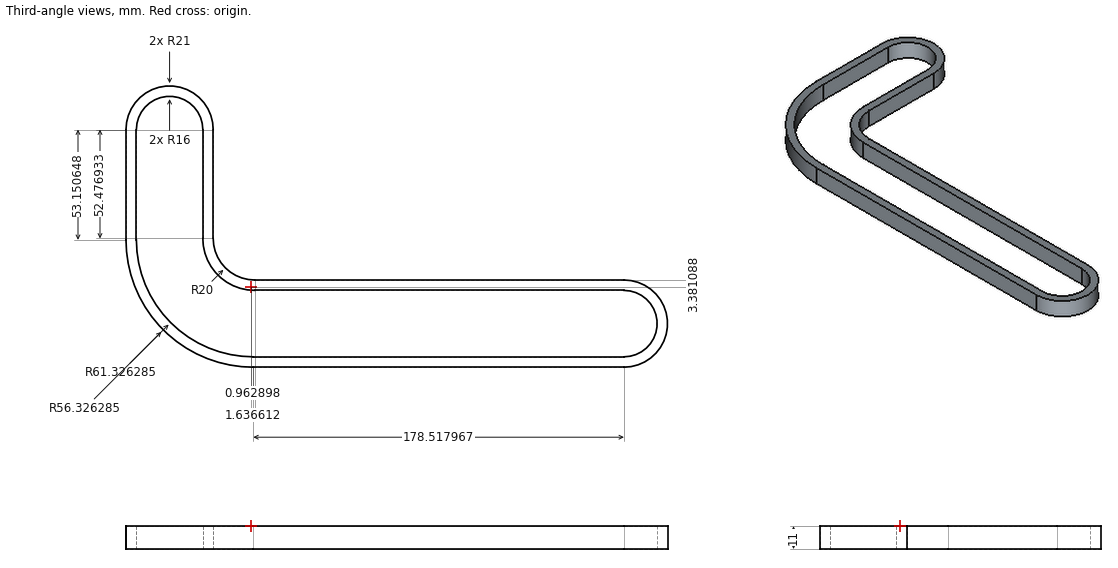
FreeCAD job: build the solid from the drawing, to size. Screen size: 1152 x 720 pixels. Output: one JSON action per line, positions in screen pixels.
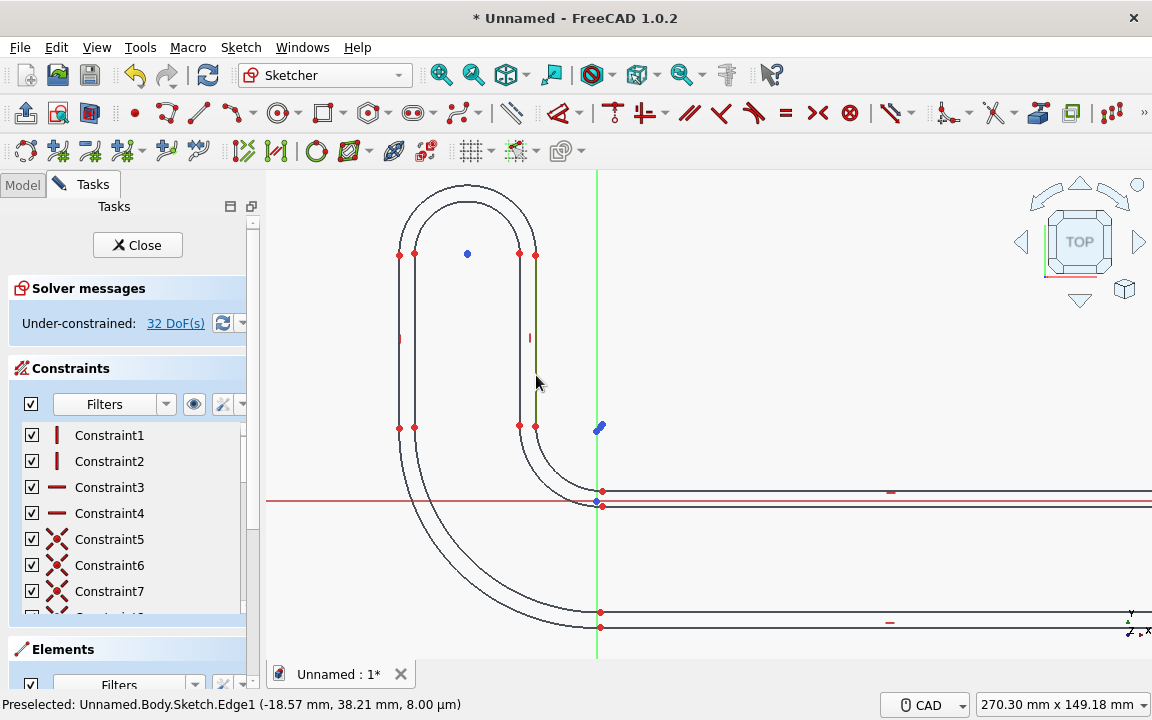
{"action": "left_click", "coordinate": [508, 199]}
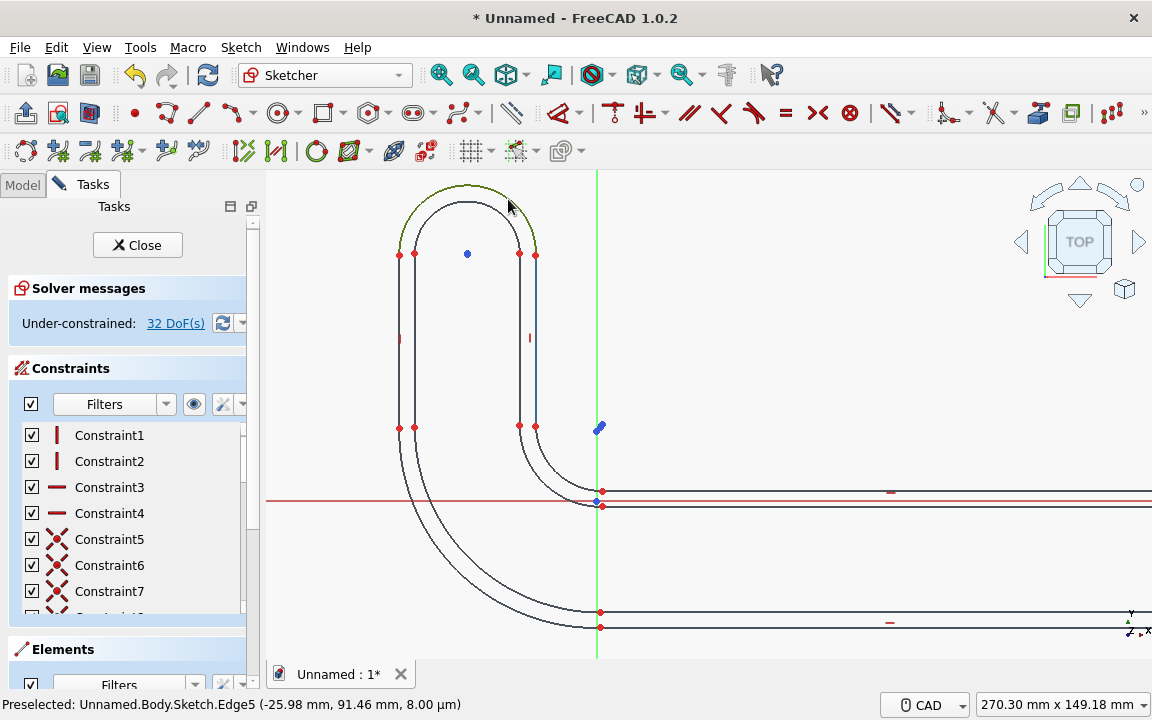
{"action": "left_click", "coordinate": [754, 114]}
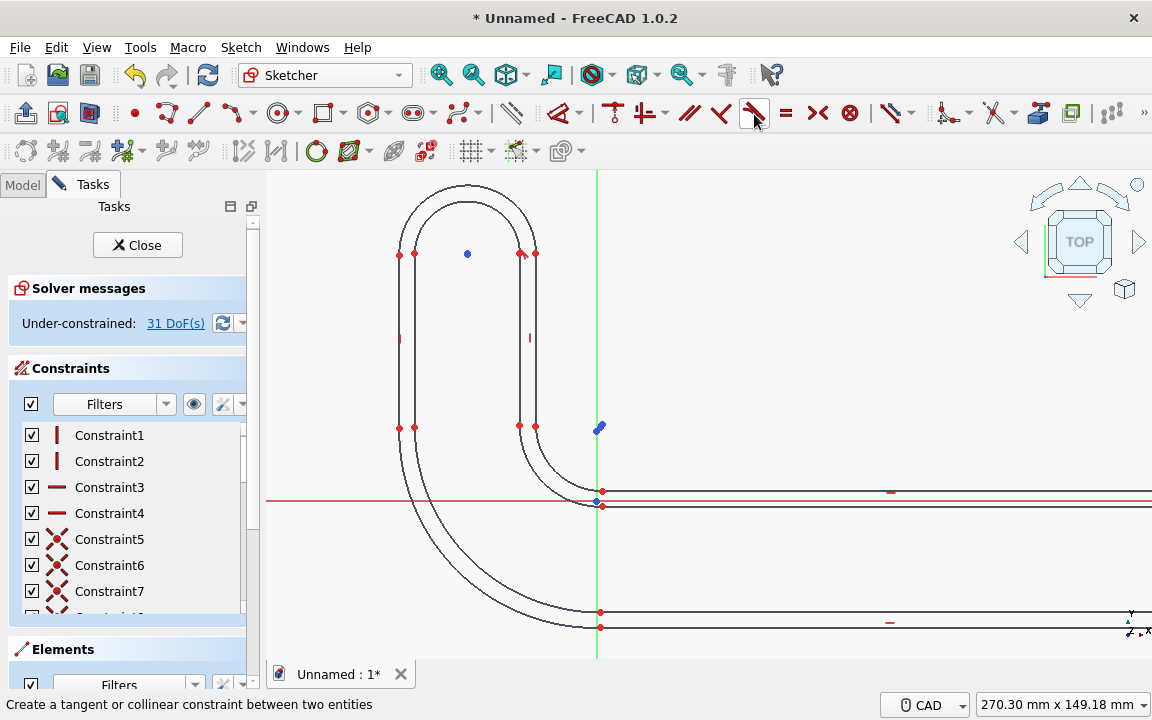
{"action": "left_click", "coordinate": [536, 375]}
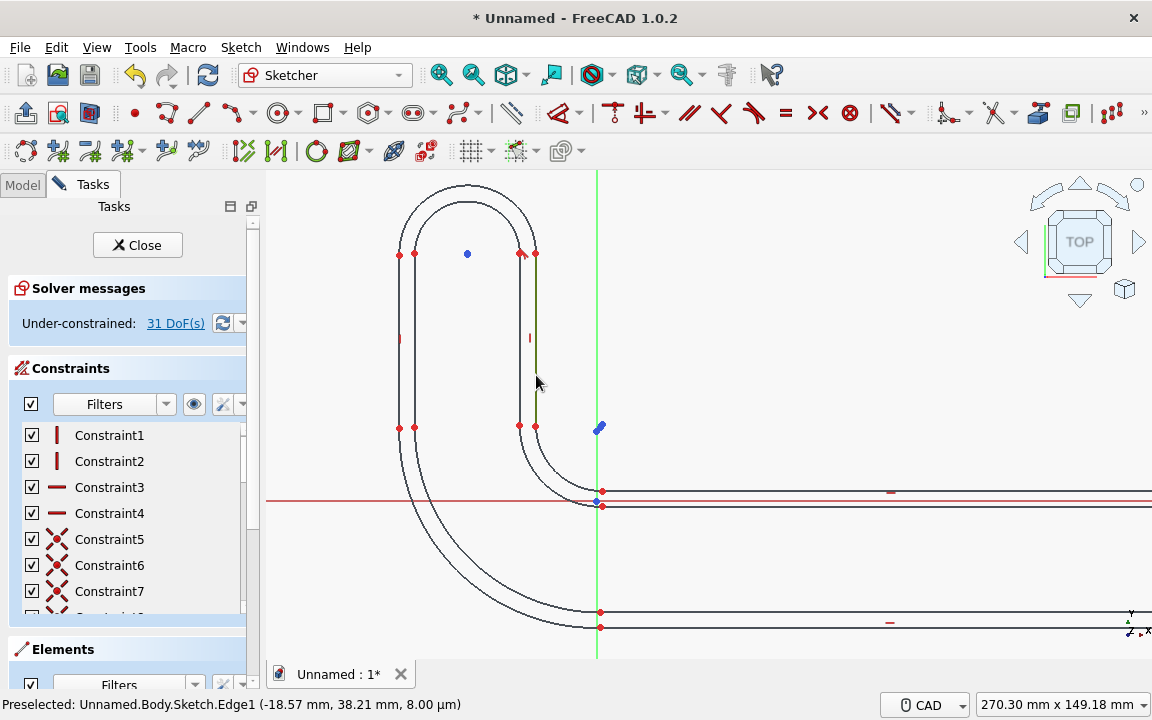
{"action": "left_click", "coordinate": [544, 456]}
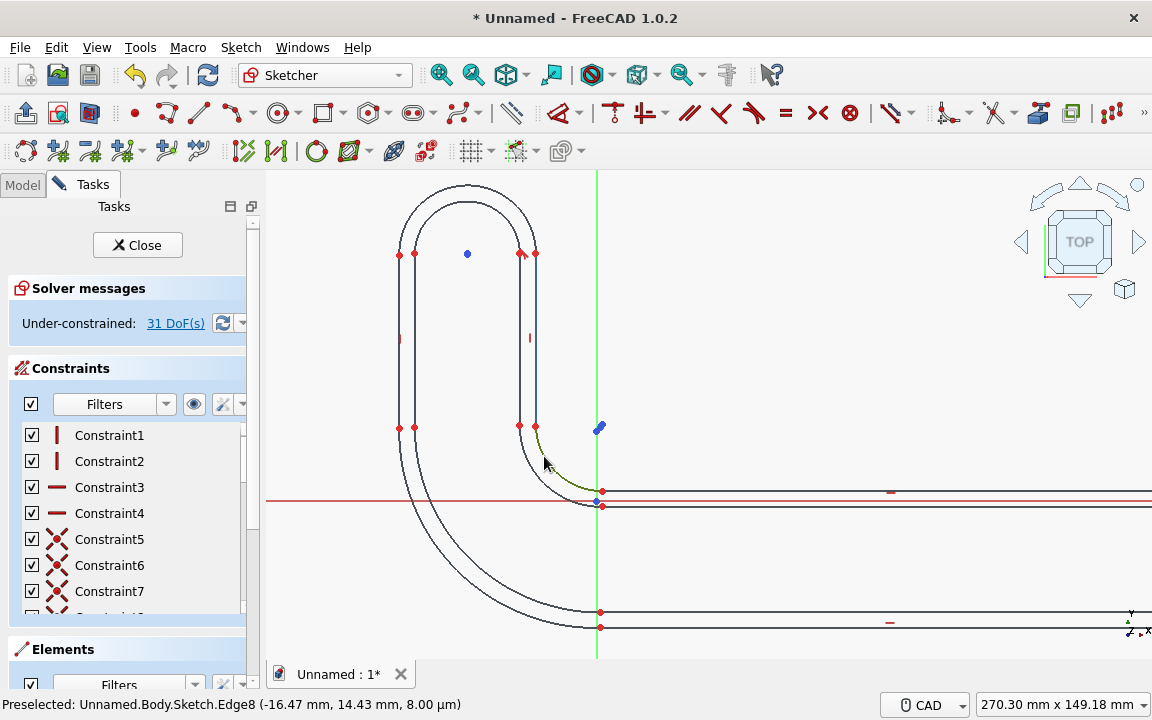
{"action": "left_click", "coordinate": [754, 114]}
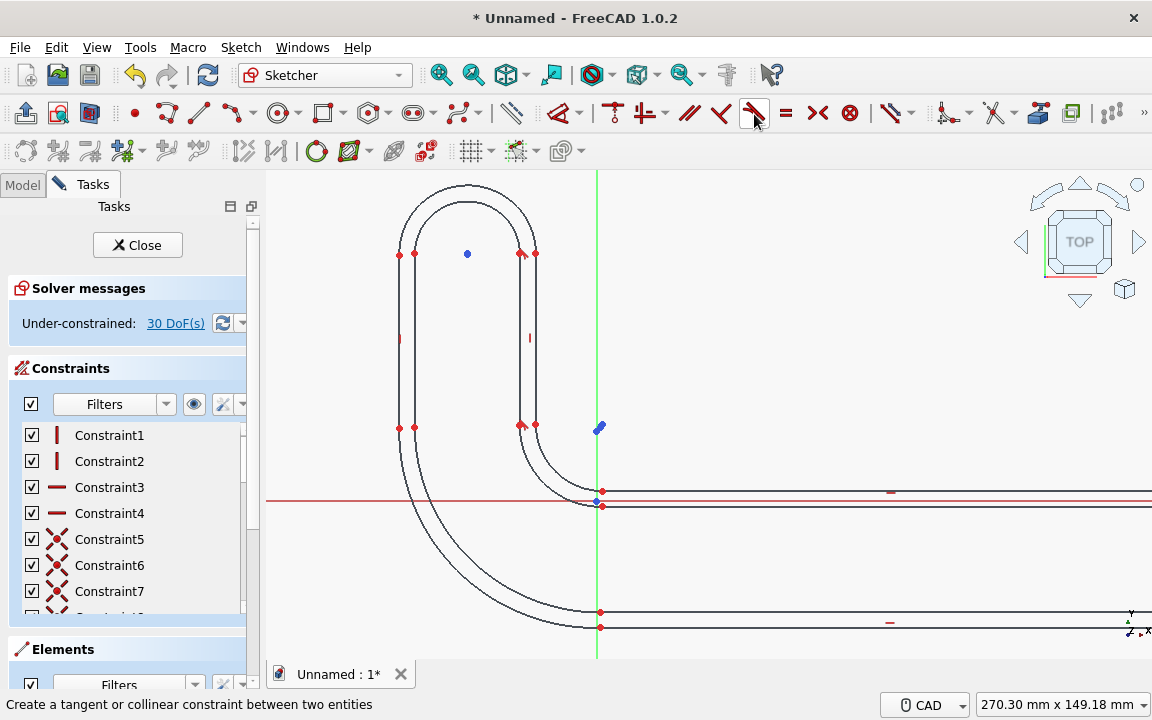
{"action": "left_click", "coordinate": [399, 307]}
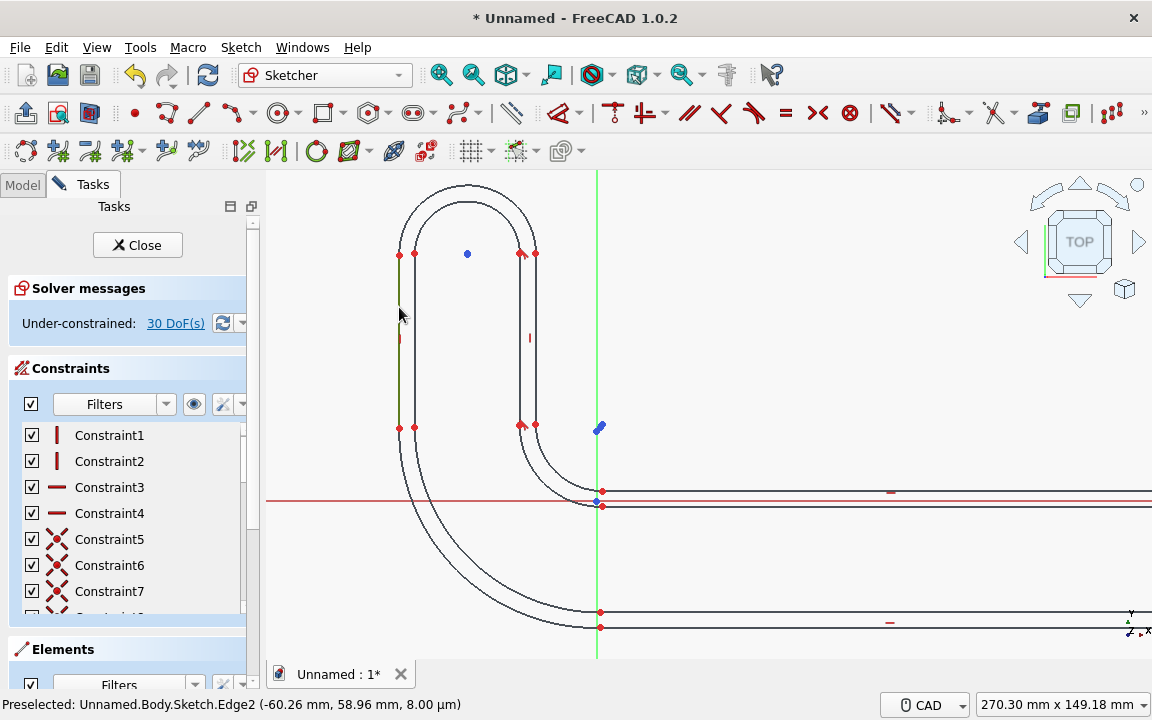
{"action": "left_click", "coordinate": [507, 198]}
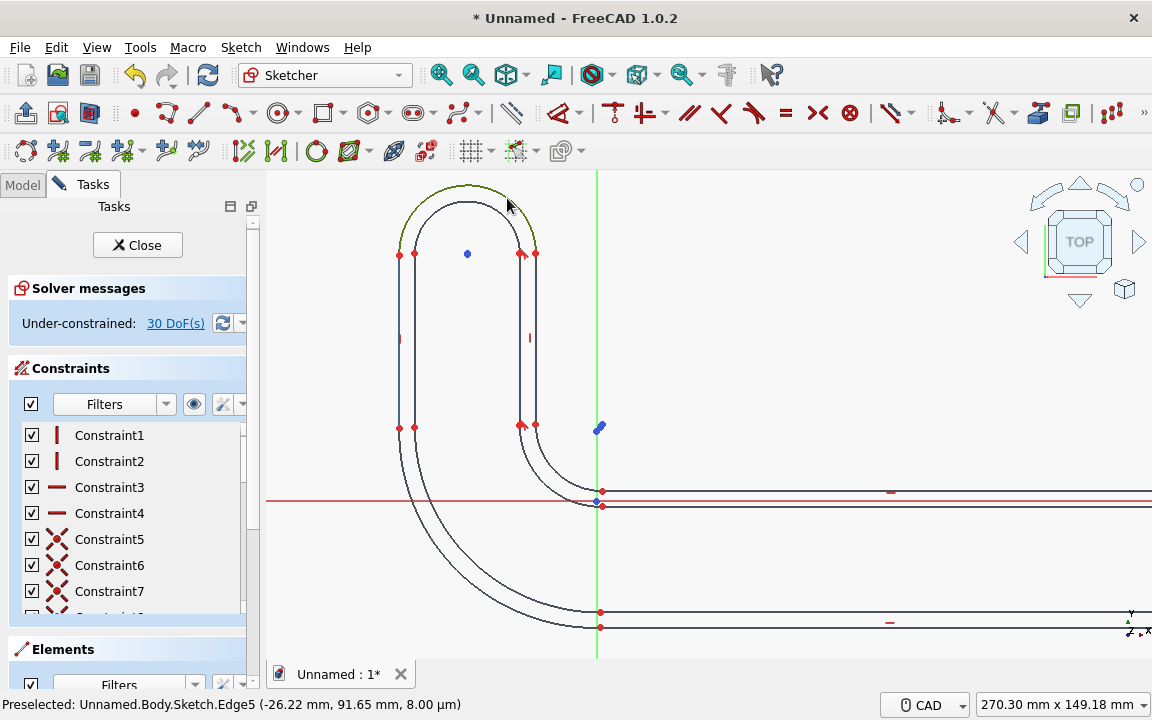
{"action": "left_click", "coordinate": [754, 114]}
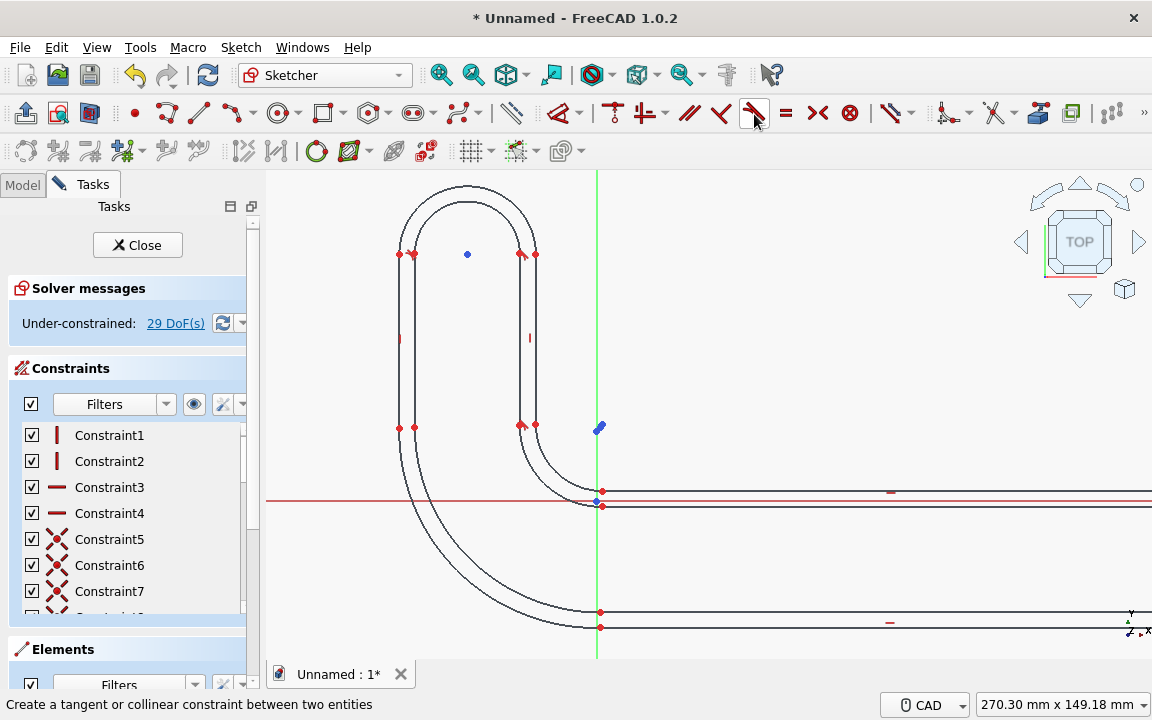
{"action": "left_click", "coordinate": [775, 628]}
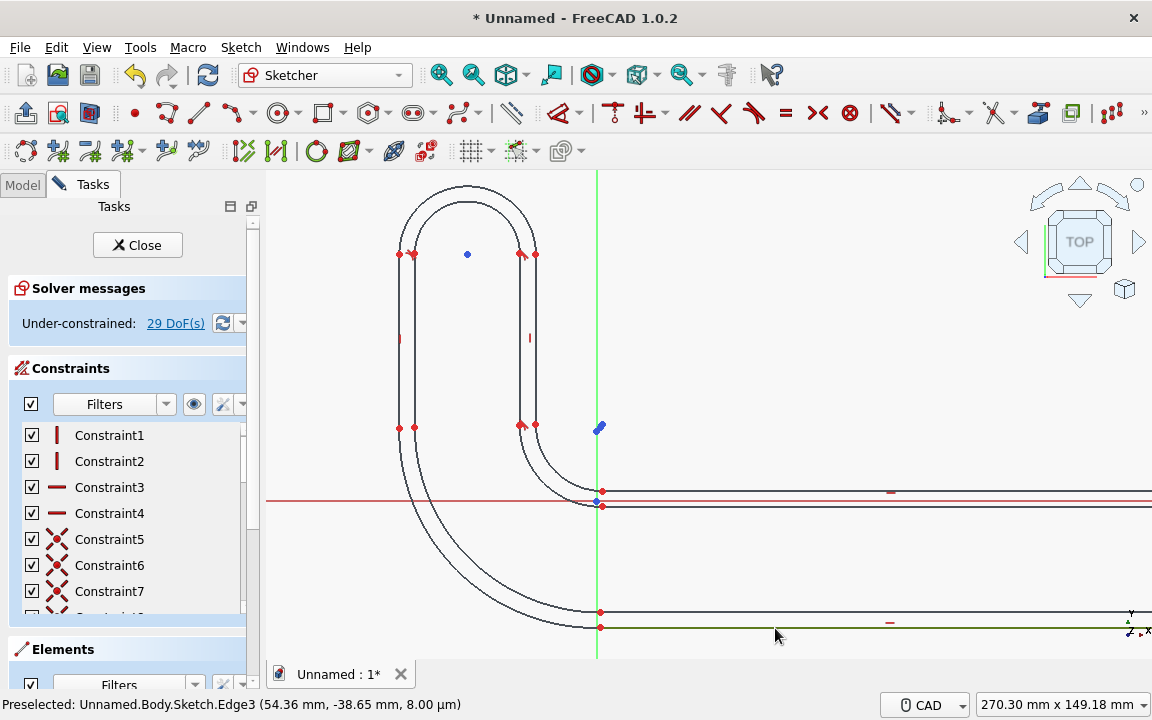
{"action": "scroll", "coordinate": [414, 425], "scroll_direction": "down", "scroll_amount": 3}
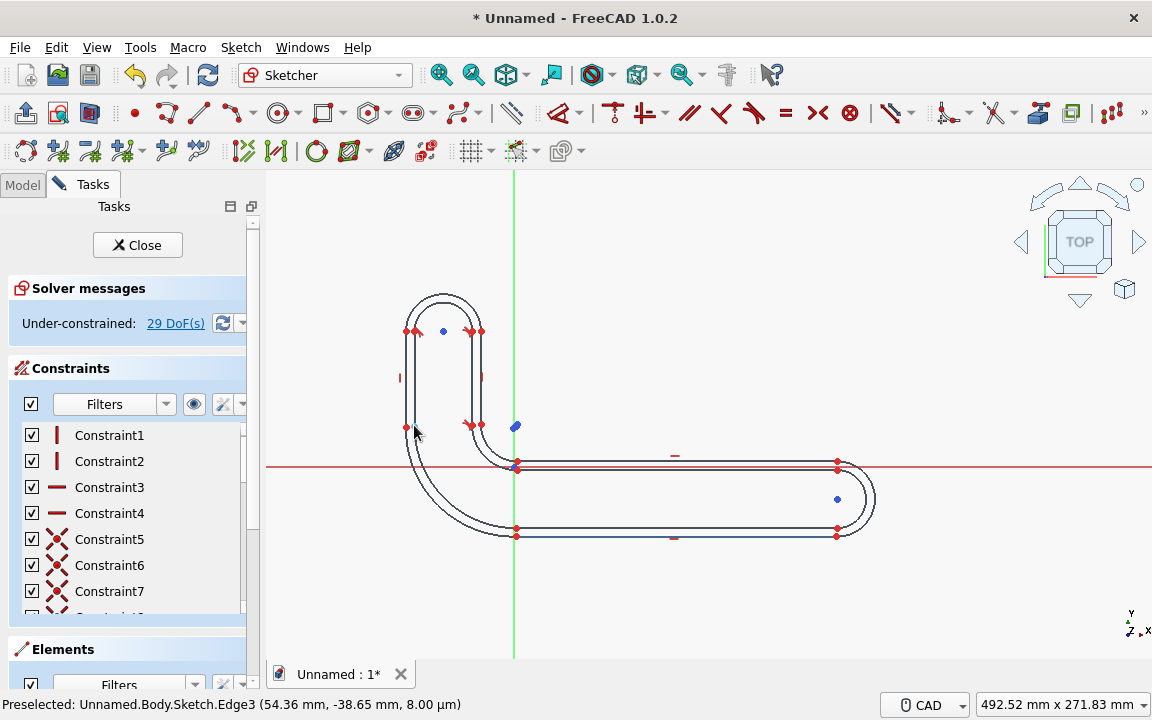
{"action": "scroll", "coordinate": [868, 521], "scroll_direction": "up", "scroll_amount": 3}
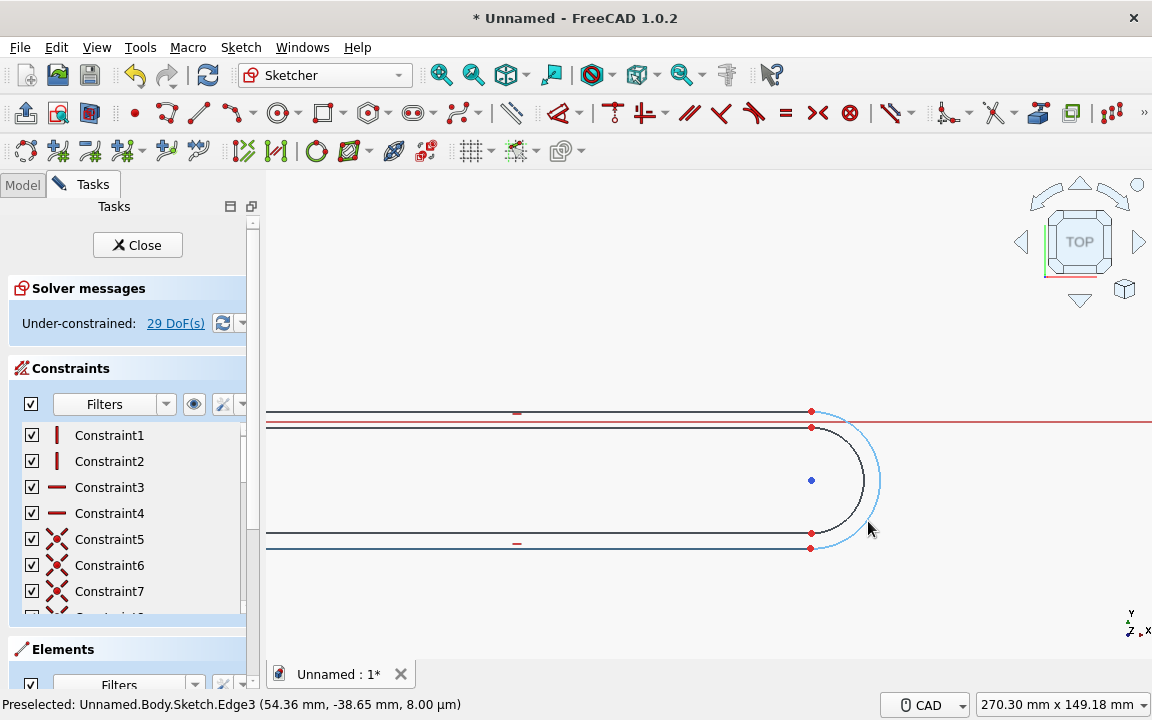
{"action": "left_click", "coordinate": [867, 521]}